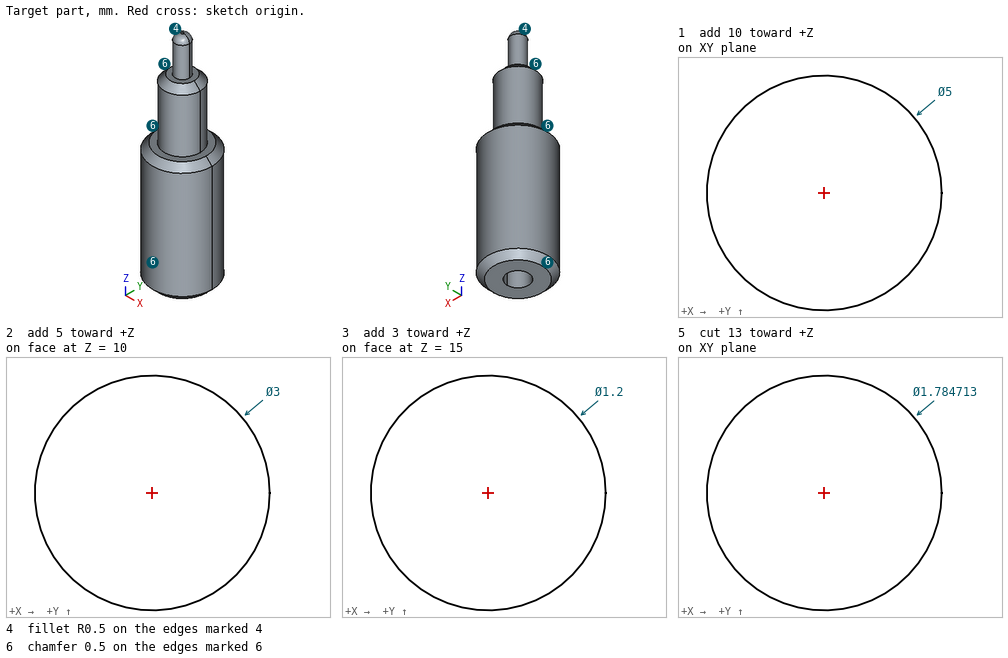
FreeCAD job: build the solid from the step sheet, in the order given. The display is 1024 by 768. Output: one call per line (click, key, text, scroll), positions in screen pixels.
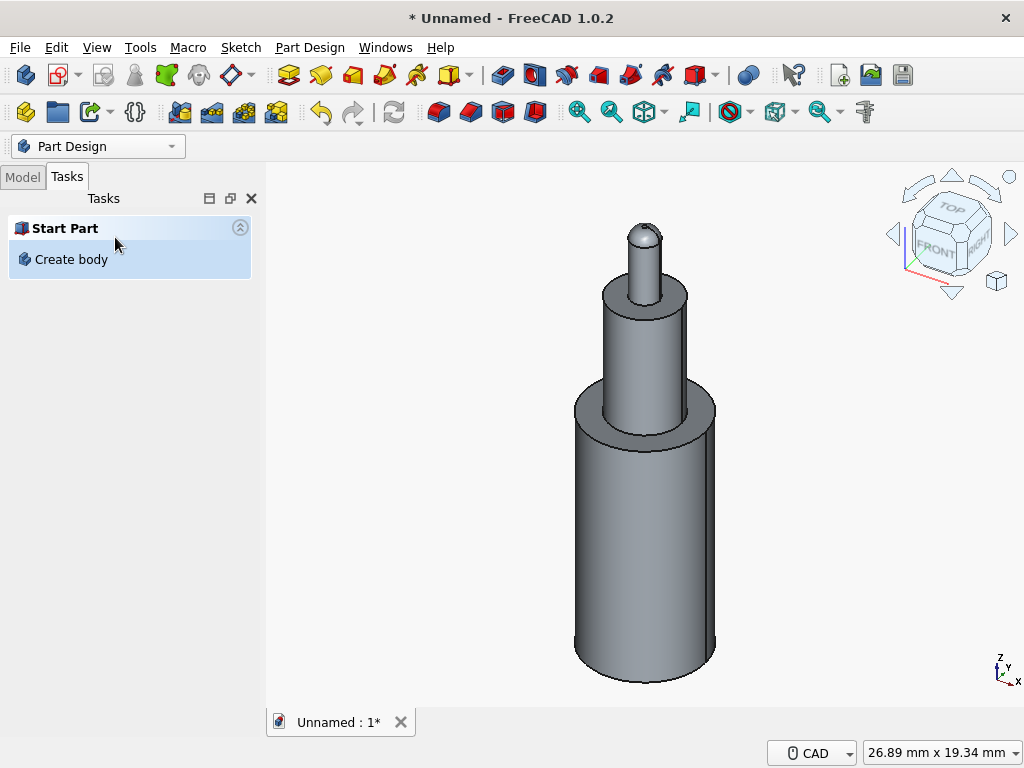
click(575, 415)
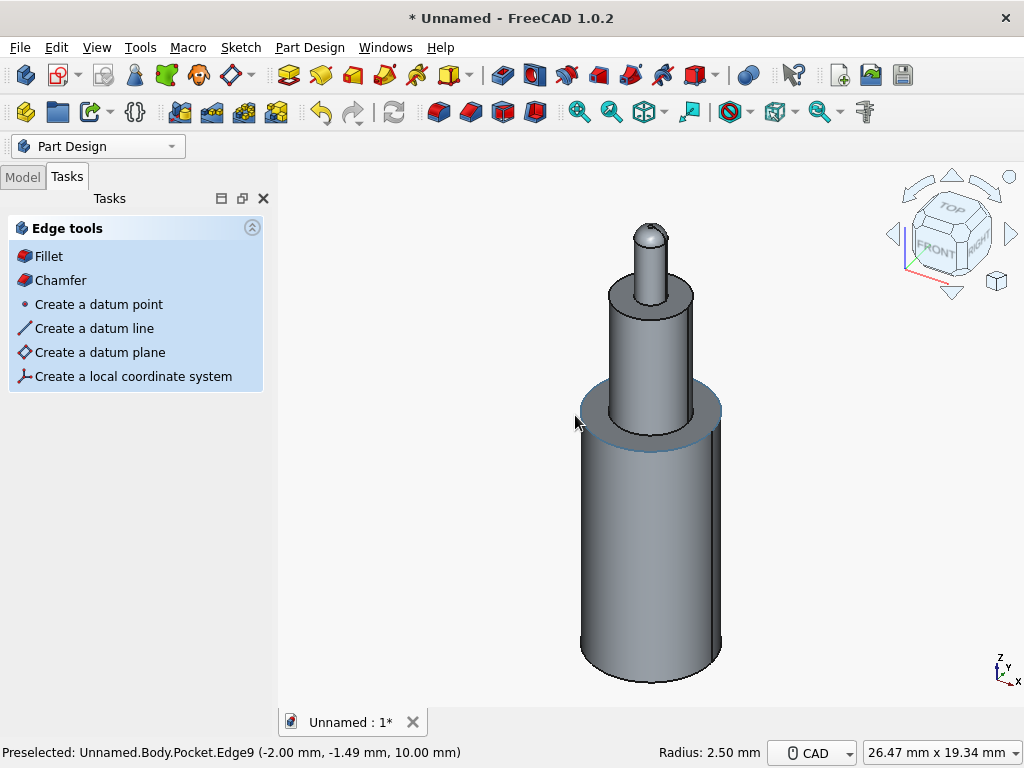
click(614, 283, ctrl)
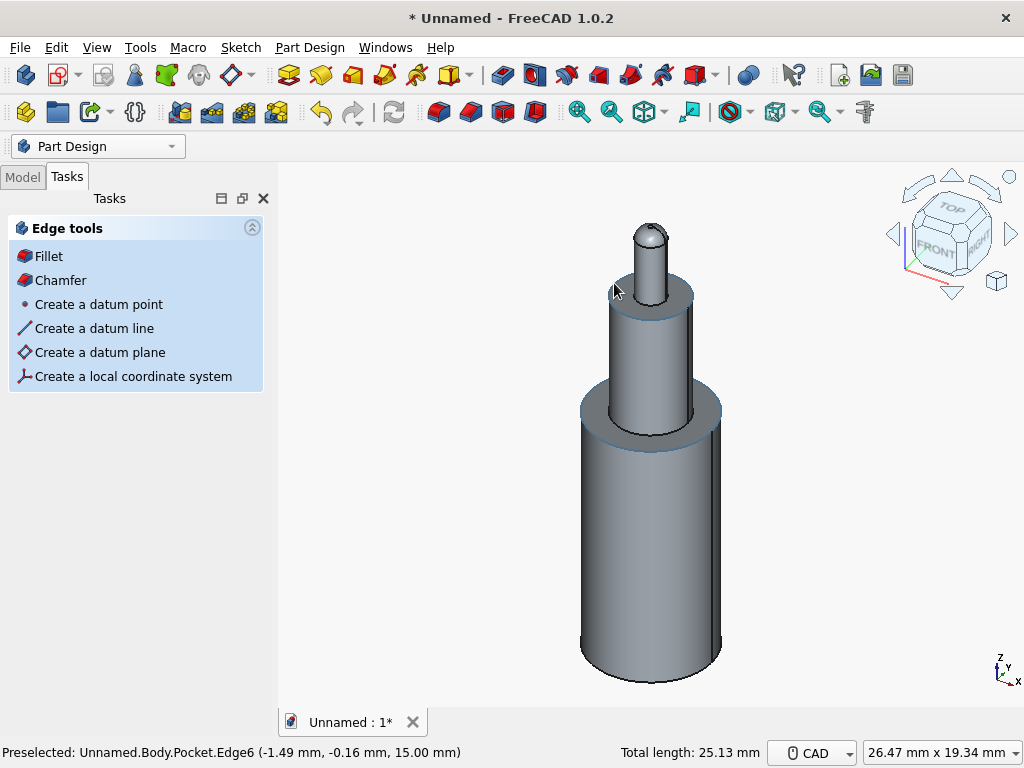
key(0)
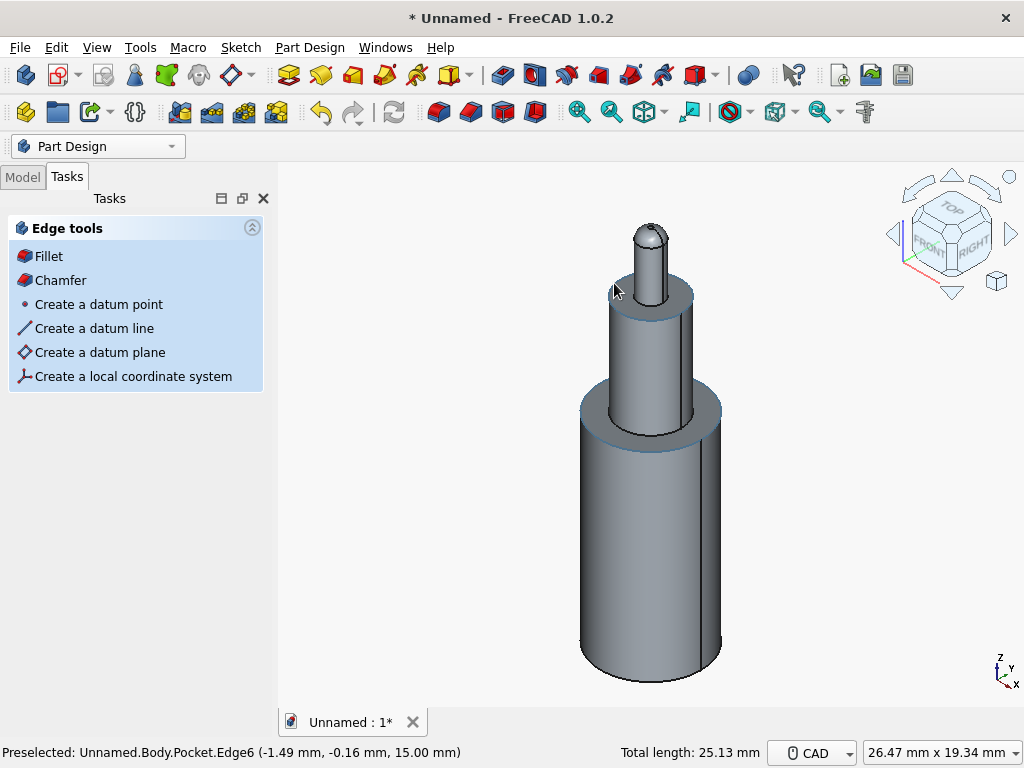
key(2)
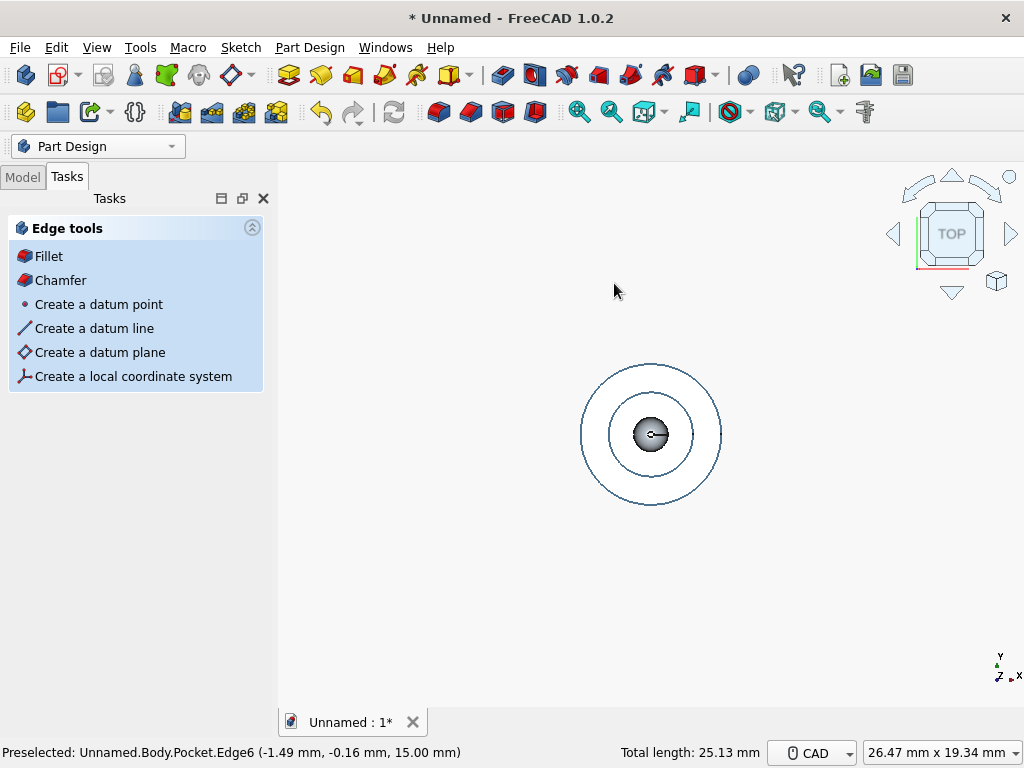
click(580, 112)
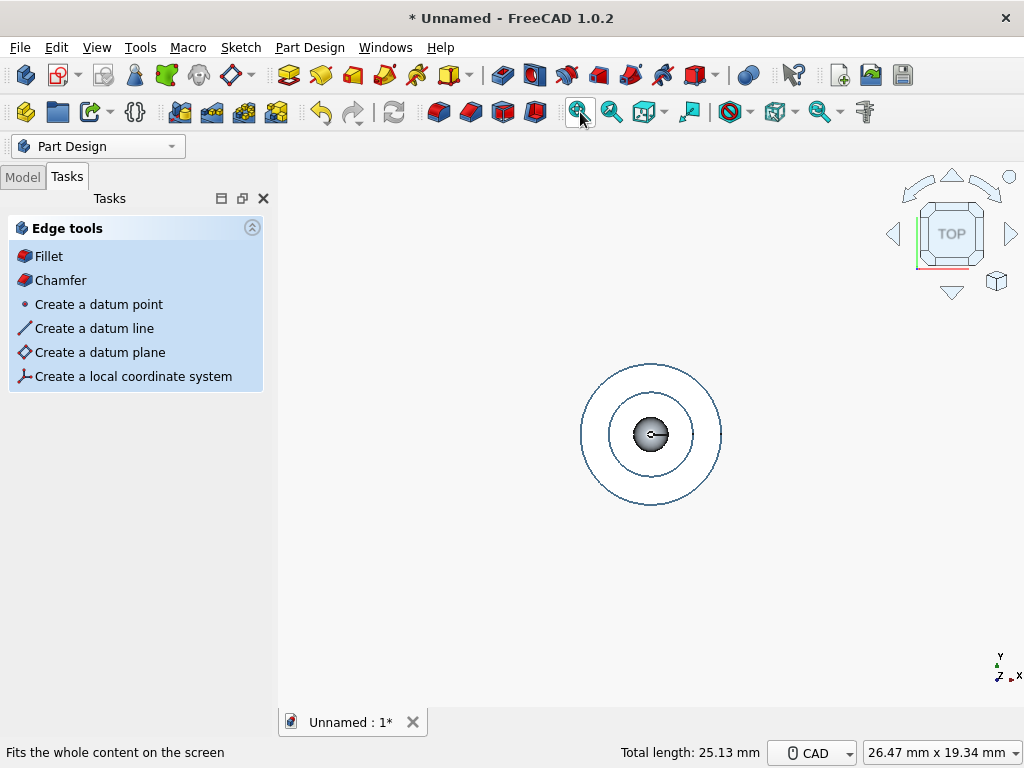
key(1)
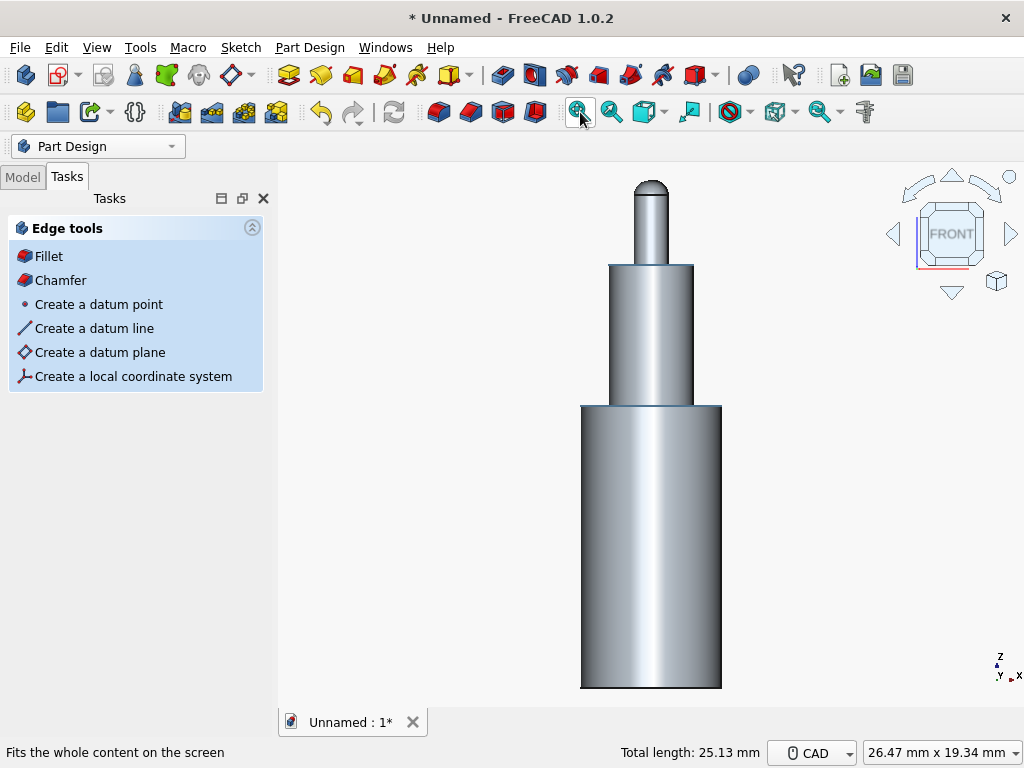
key(3)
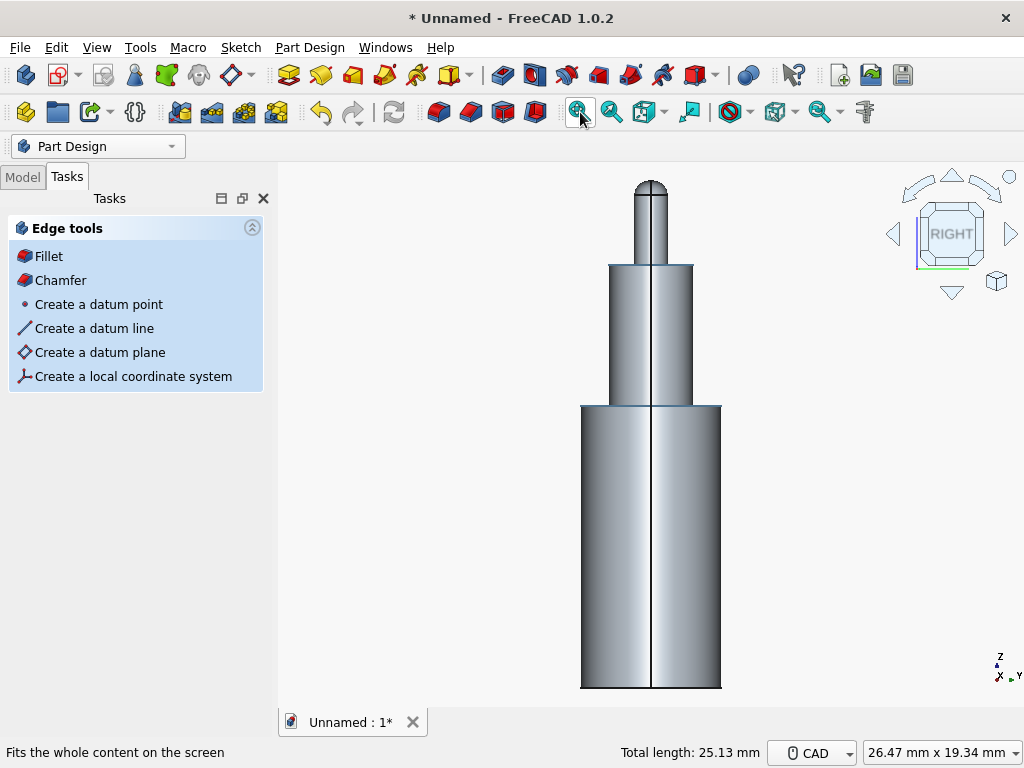
key(5)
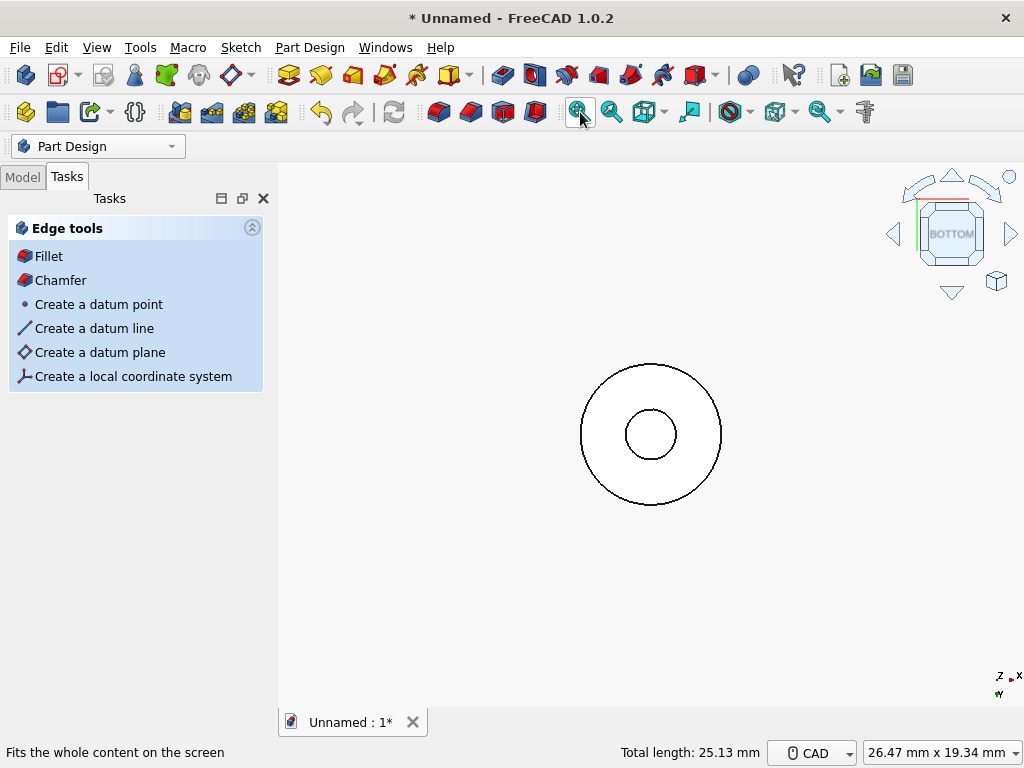
click(580, 112)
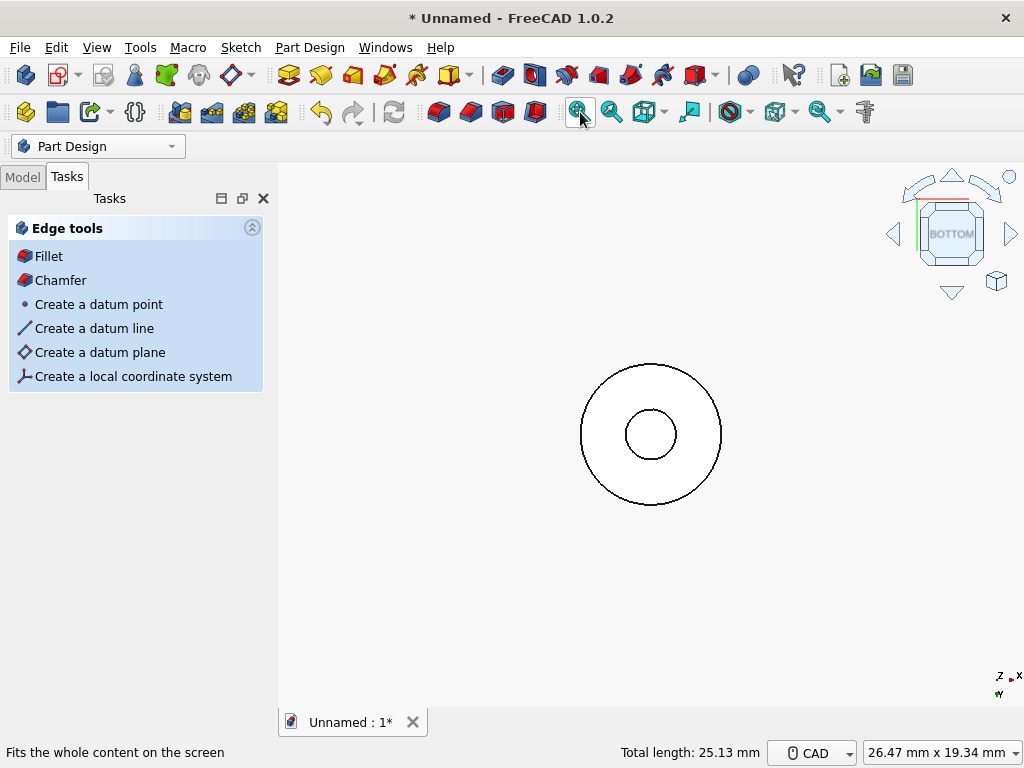
click(580, 433, ctrl)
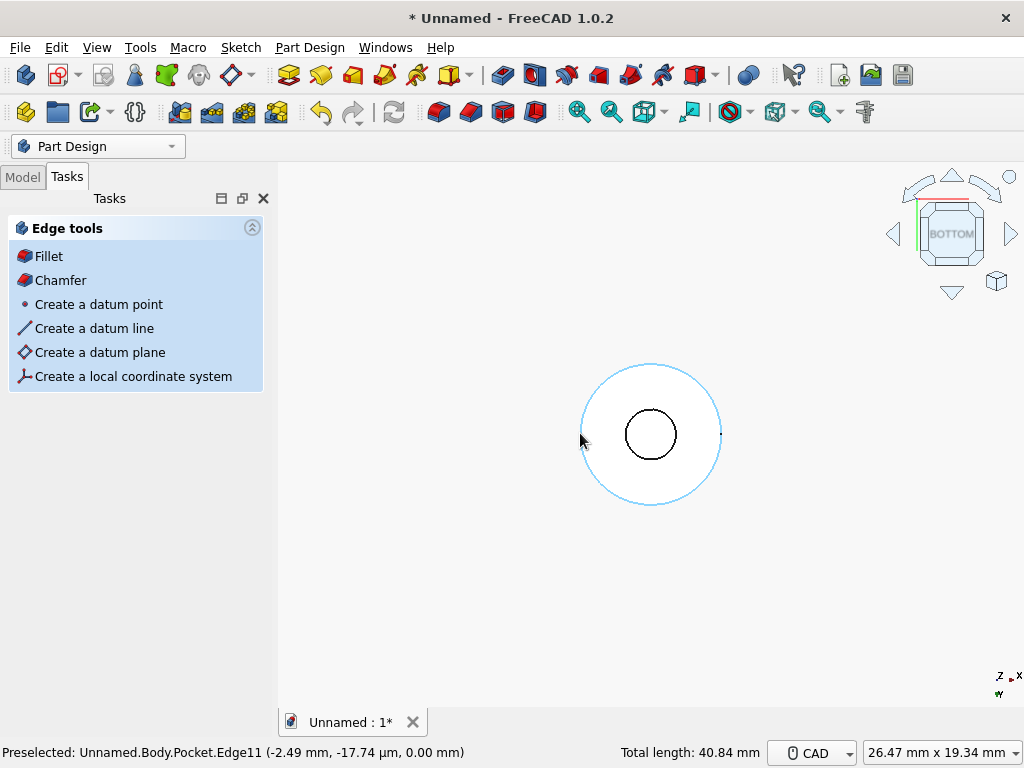
click(472, 112)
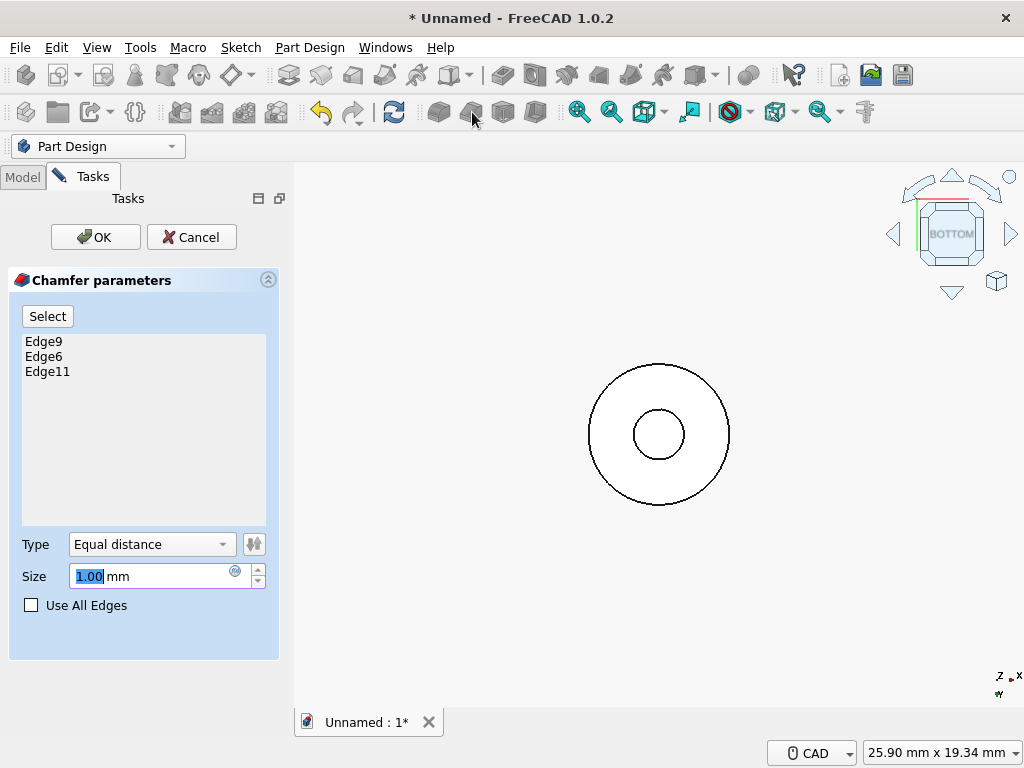
text(0.5)
key(Tab)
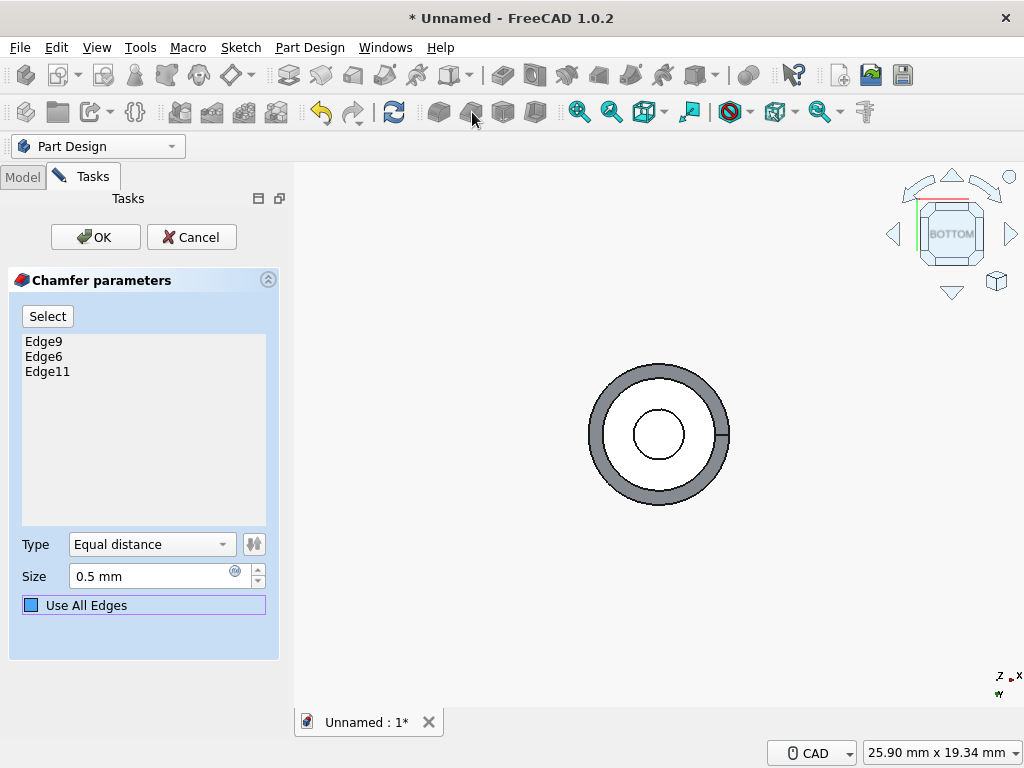
click(96, 237)